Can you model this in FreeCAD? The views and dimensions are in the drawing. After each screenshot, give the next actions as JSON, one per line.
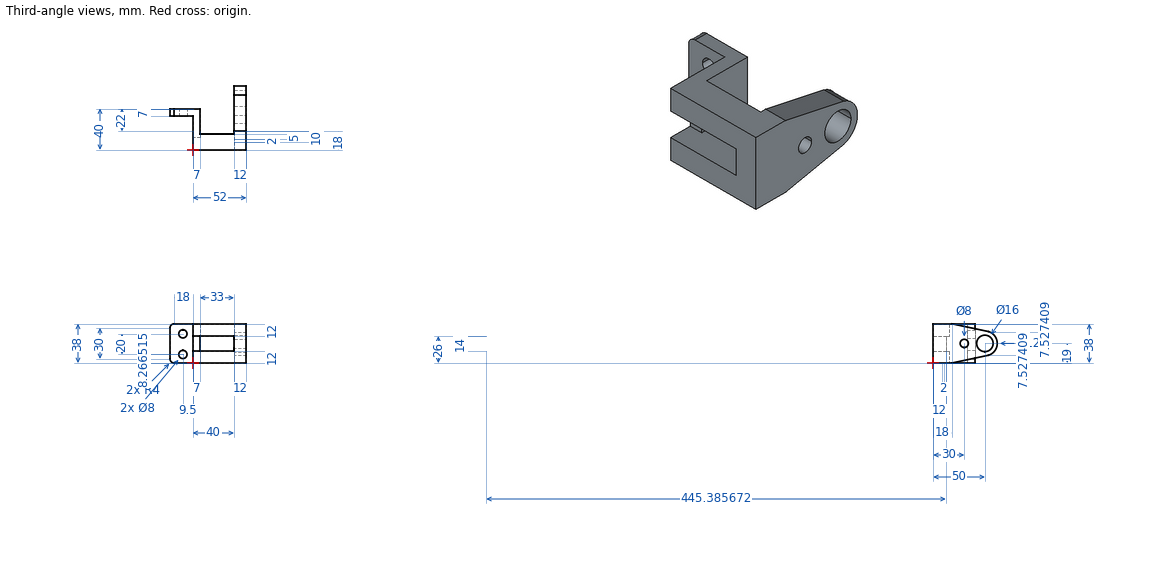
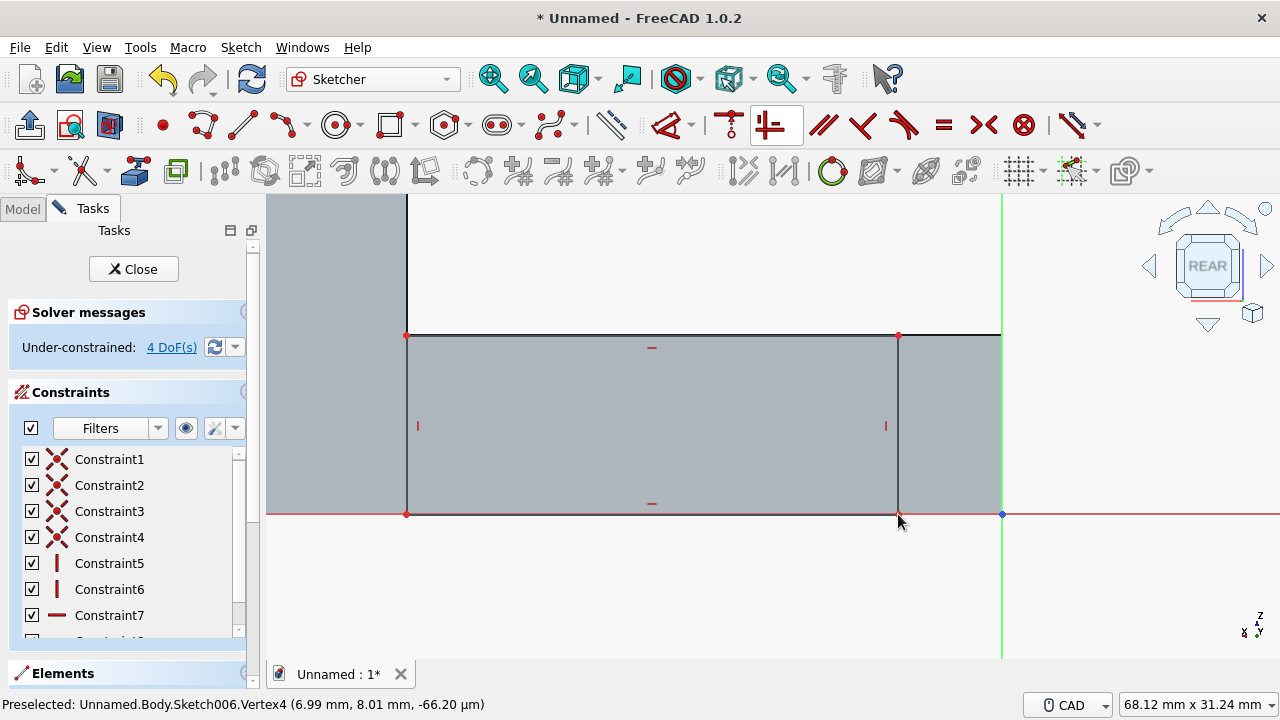
{"action": "left_click", "coordinate": [407, 515]}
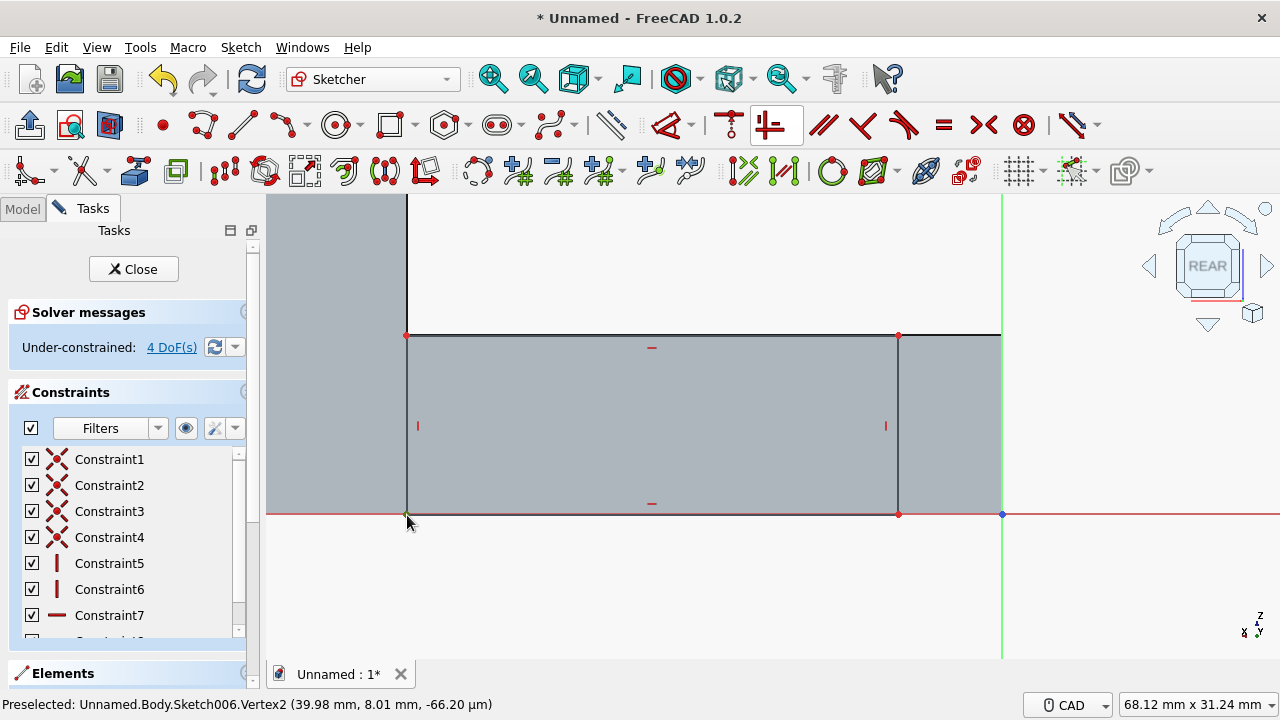
{"action": "left_click", "coordinate": [353, 514]}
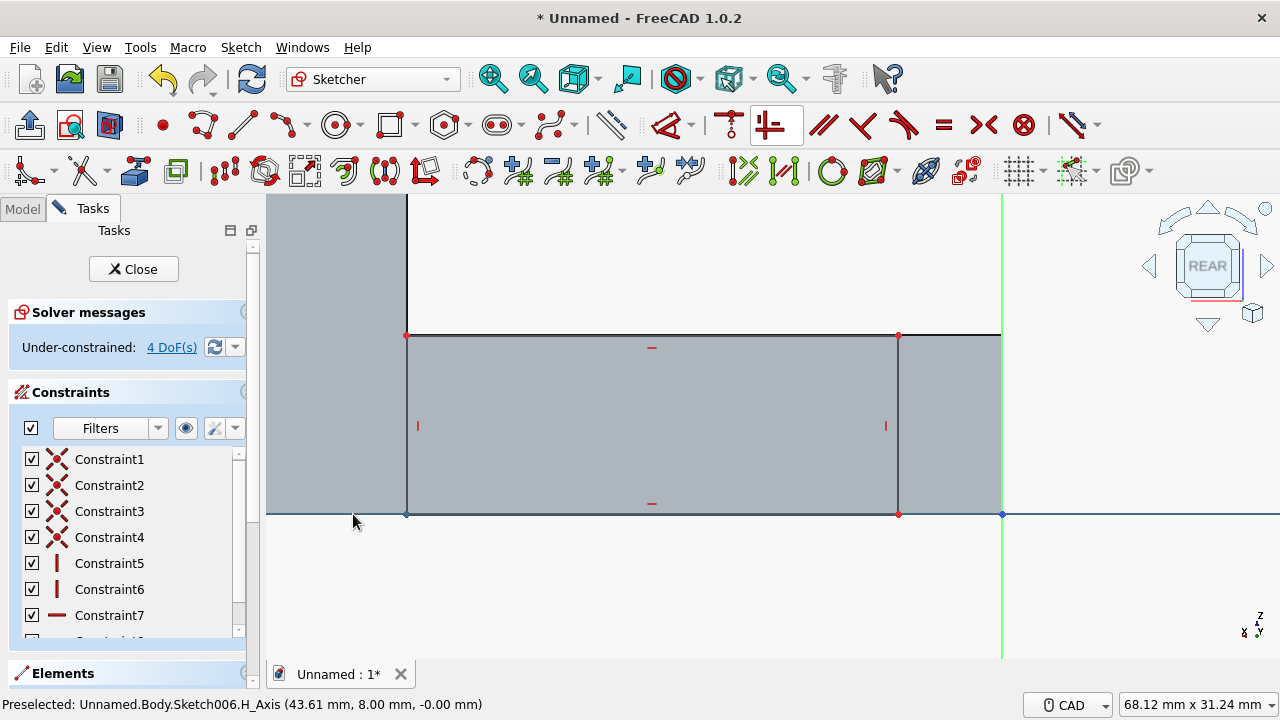
{"action": "left_click", "coordinate": [730, 126]}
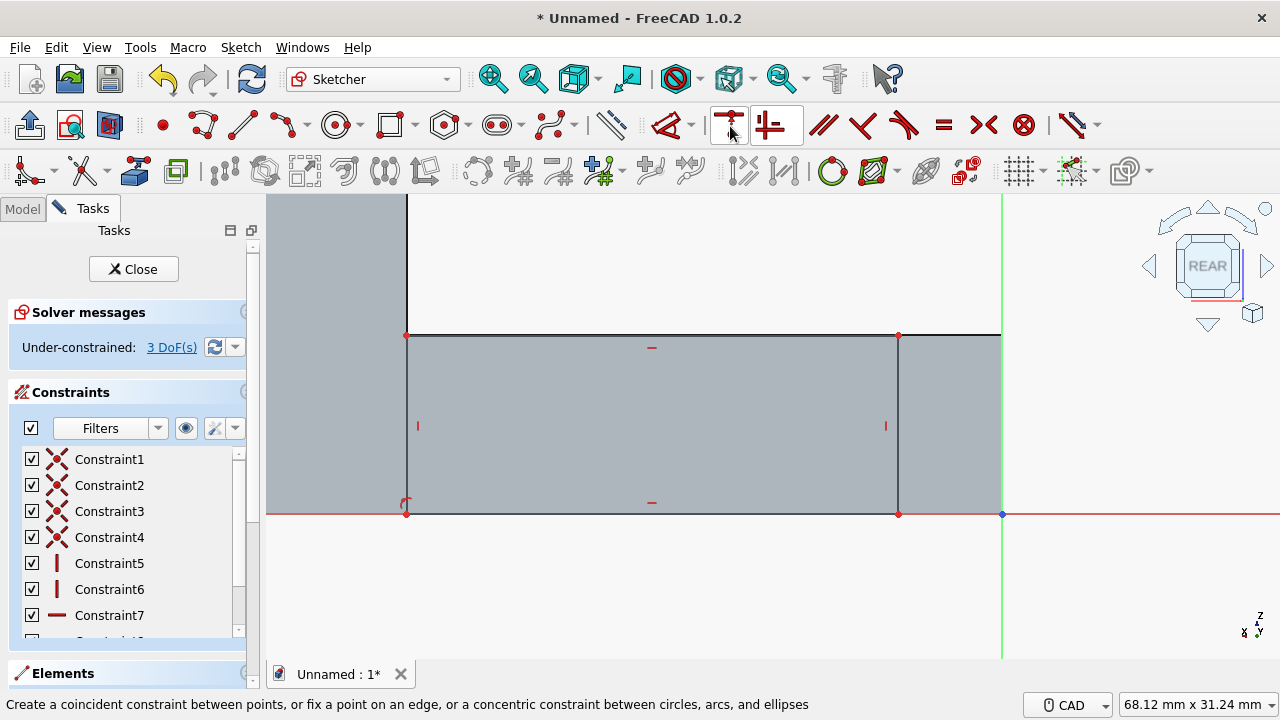
{"action": "left_click", "coordinate": [666, 126]}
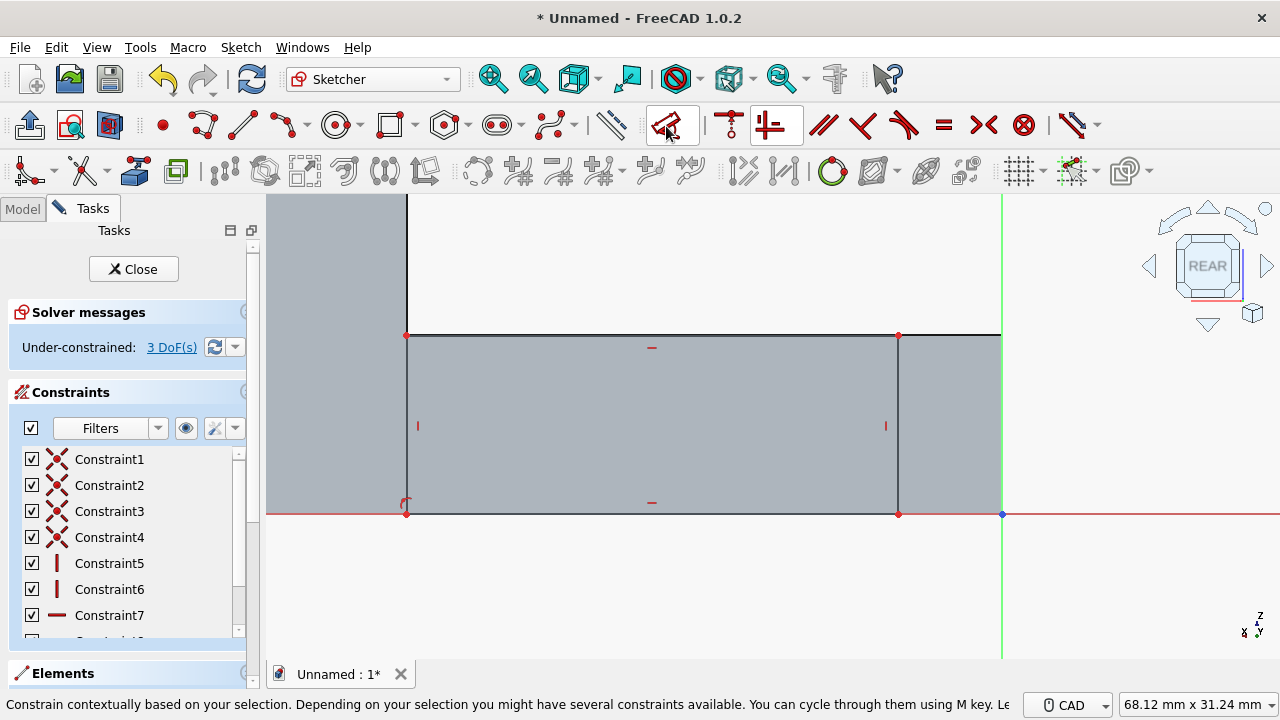
{"action": "left_click", "coordinate": [407, 389]}
{"action": "left_click", "coordinate": [373, 425]}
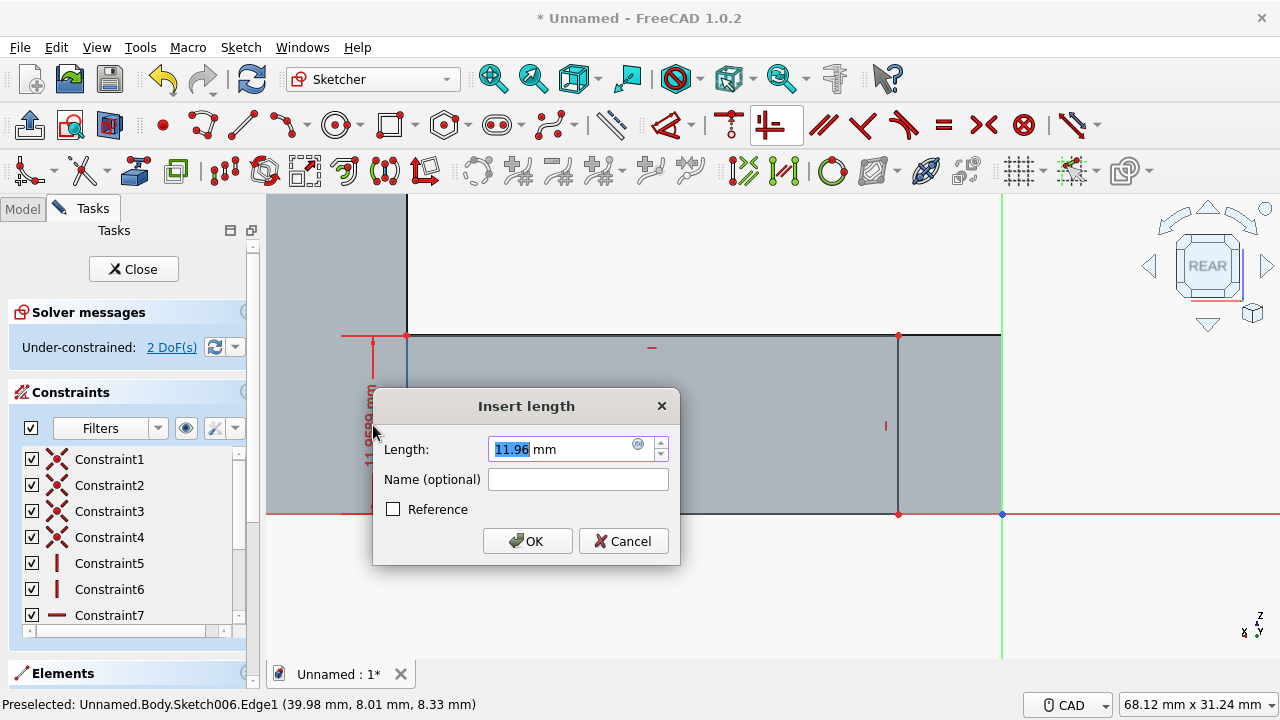
{"action": "type", "text": "12"}
{"action": "key", "text": "Return"}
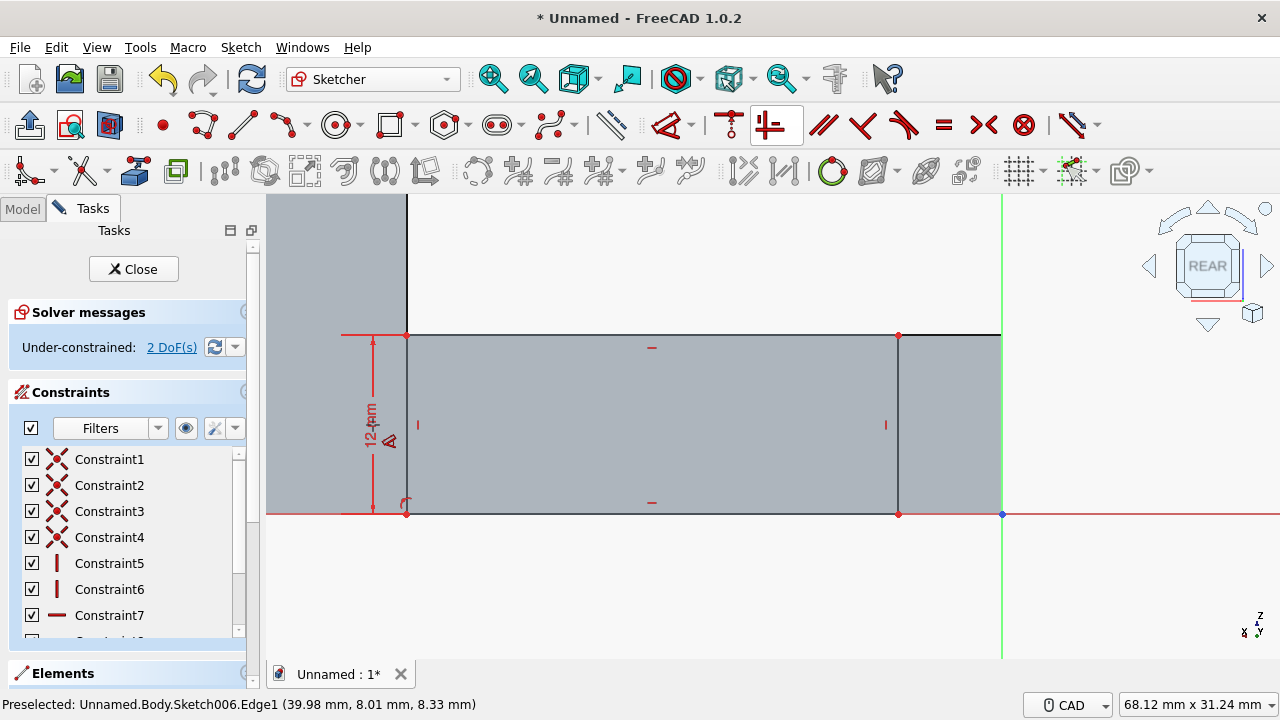
{"action": "left_click", "coordinate": [554, 514]}
{"action": "left_click", "coordinate": [652, 548]}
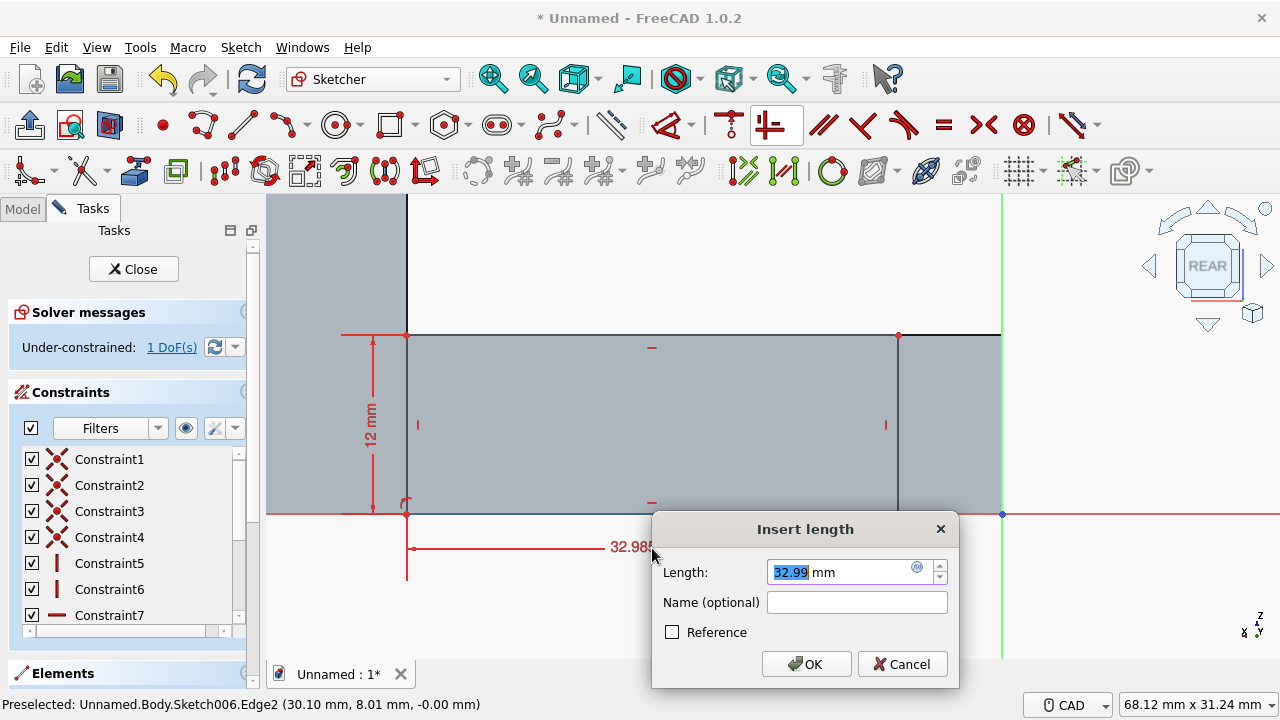
{"action": "type", "text": "33"}
{"action": "key", "text": "Return"}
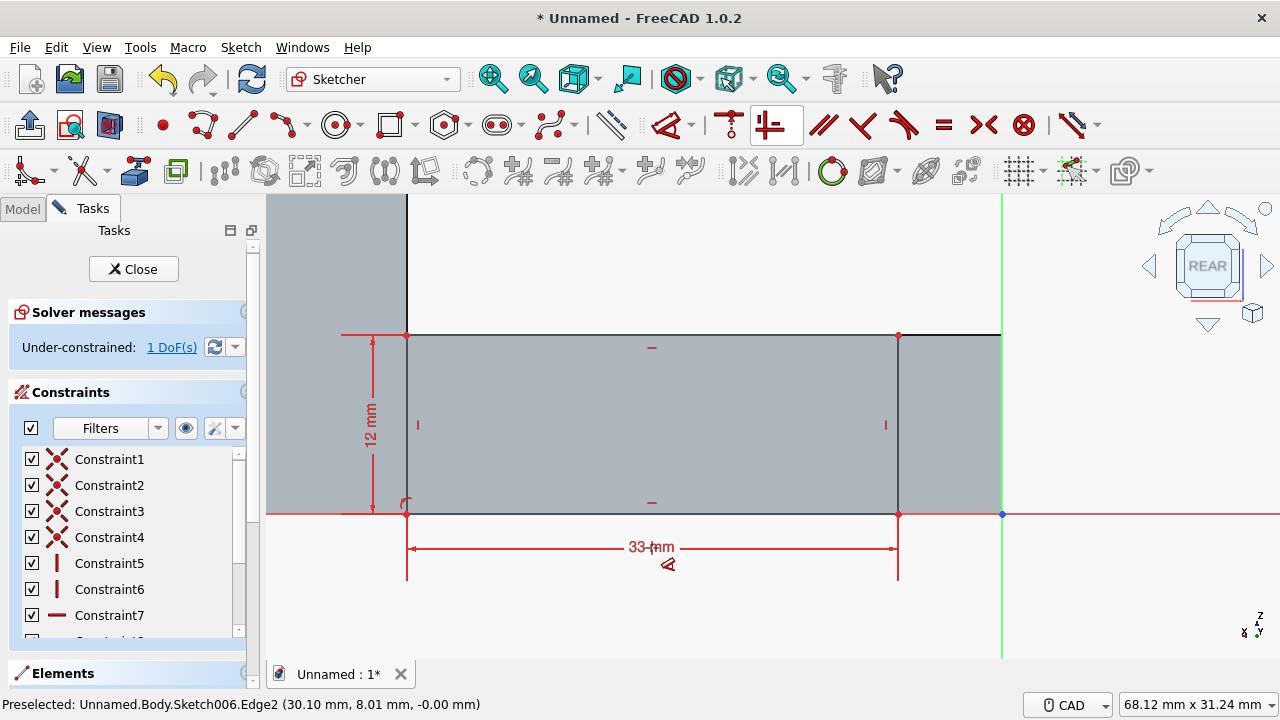
{"action": "left_click", "coordinate": [898, 514]}
{"action": "left_click", "coordinate": [950, 548]}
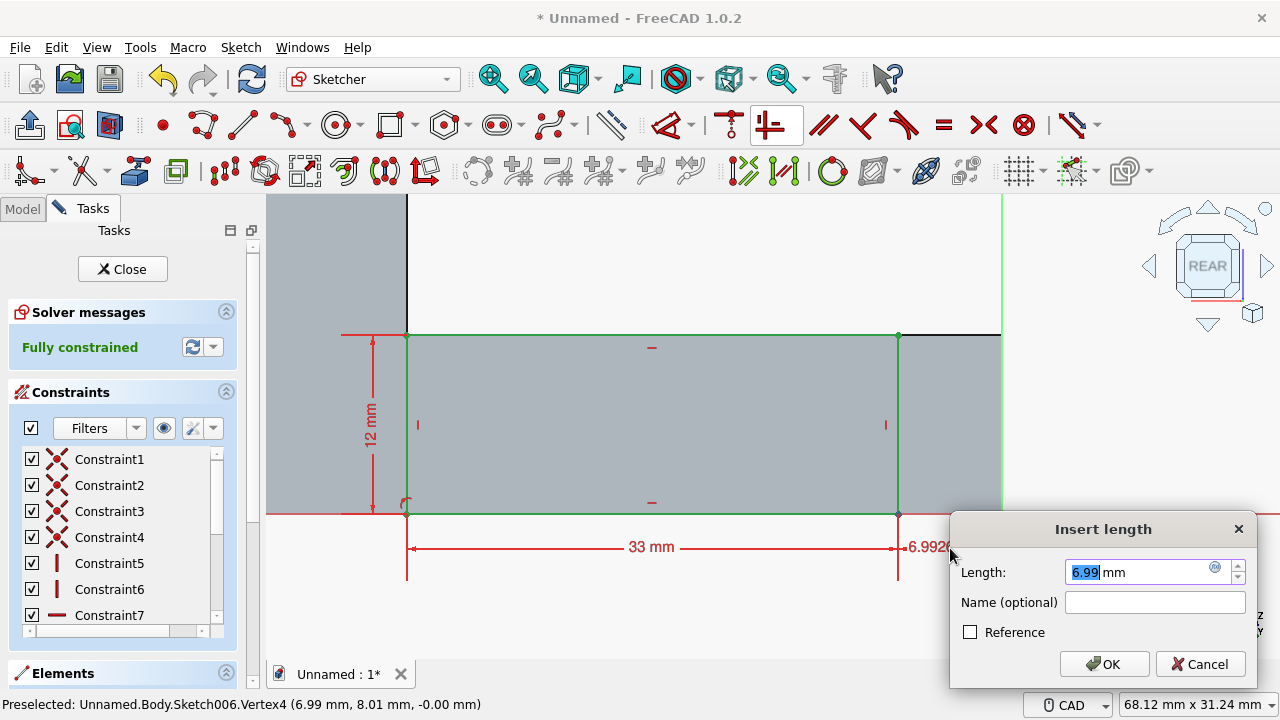
{"action": "type", "text": "7"}
{"action": "key", "text": "Return"}
{"action": "key", "text": "Escape"}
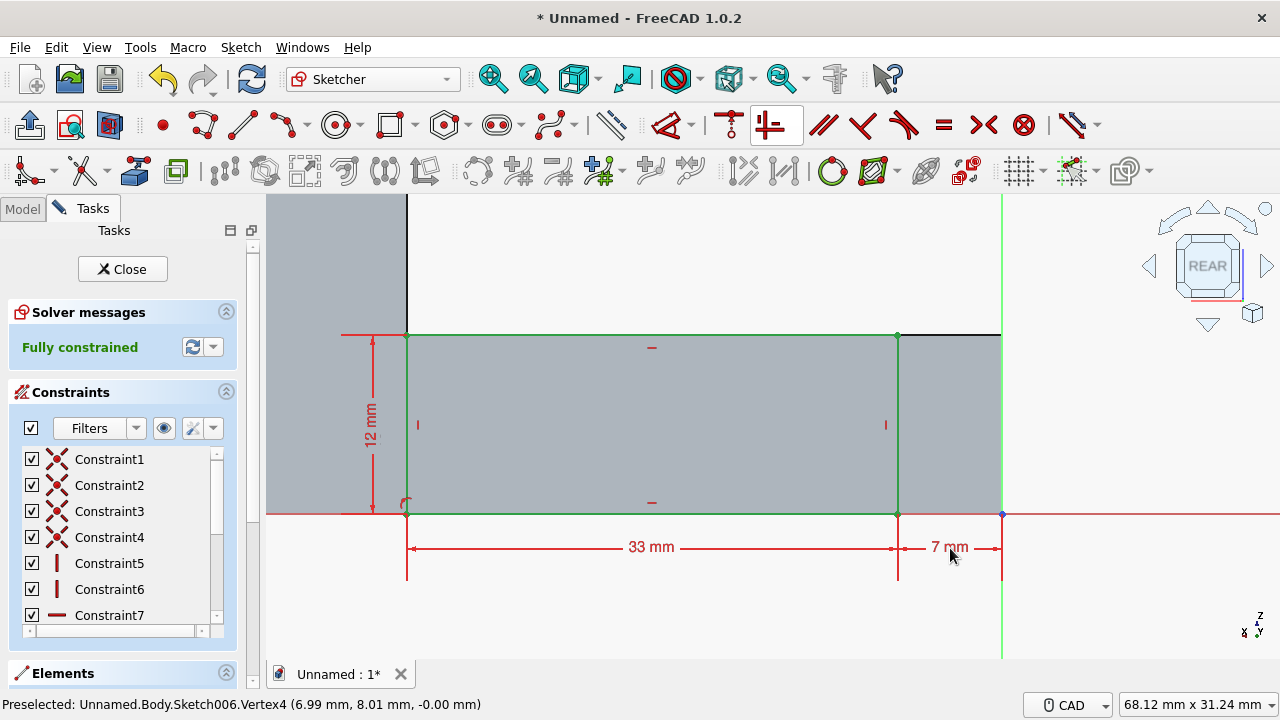
{"action": "left_click", "coordinate": [123, 269]}